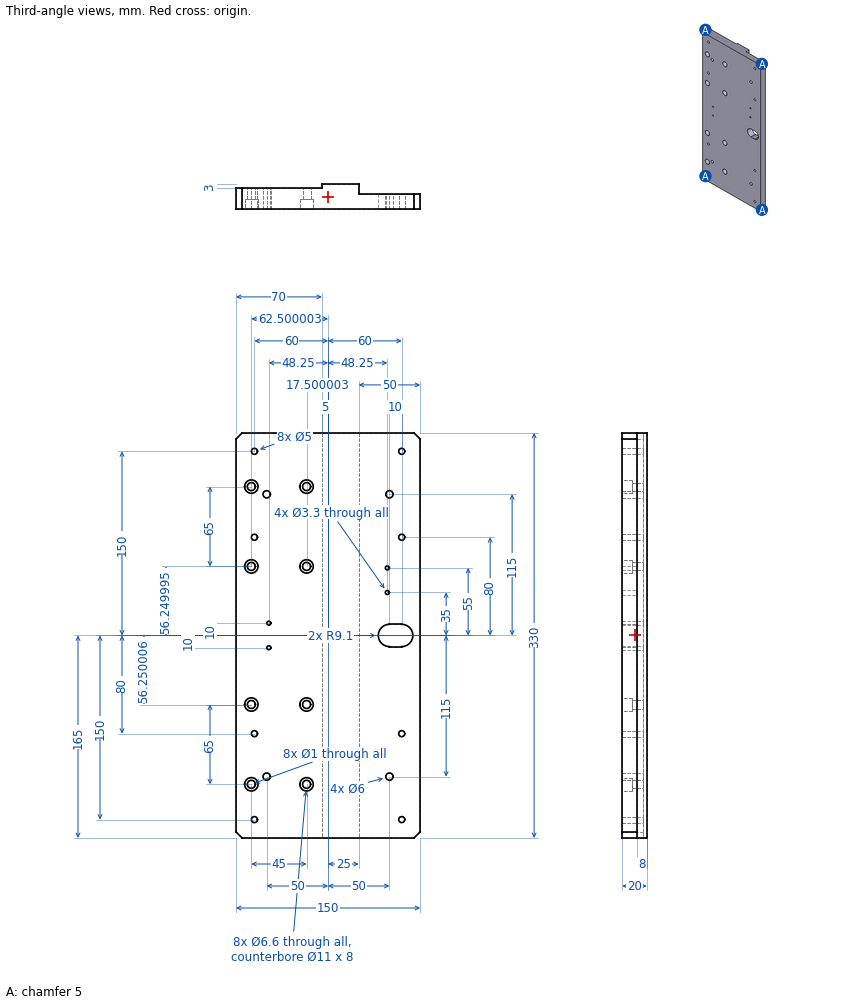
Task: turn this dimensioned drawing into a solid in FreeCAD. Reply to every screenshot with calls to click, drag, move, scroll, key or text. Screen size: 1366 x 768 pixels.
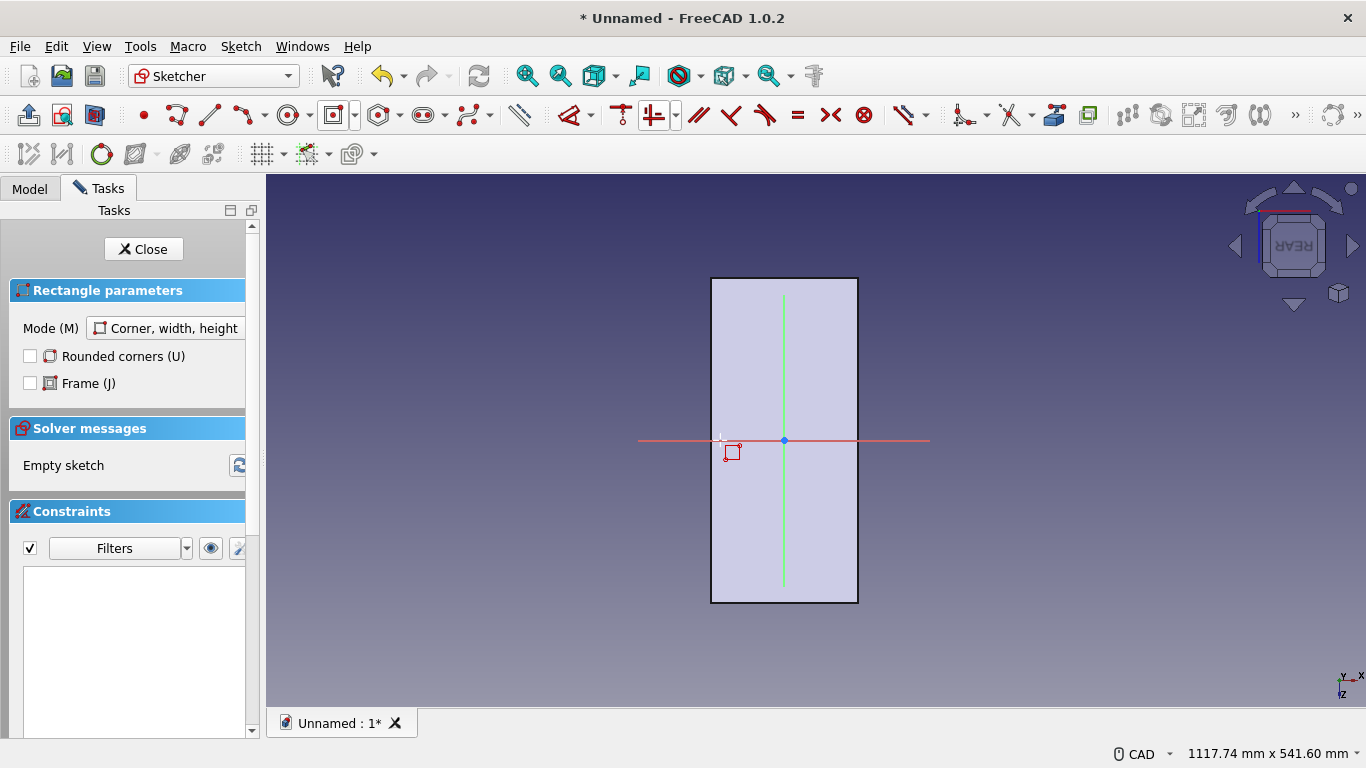
click(711, 278)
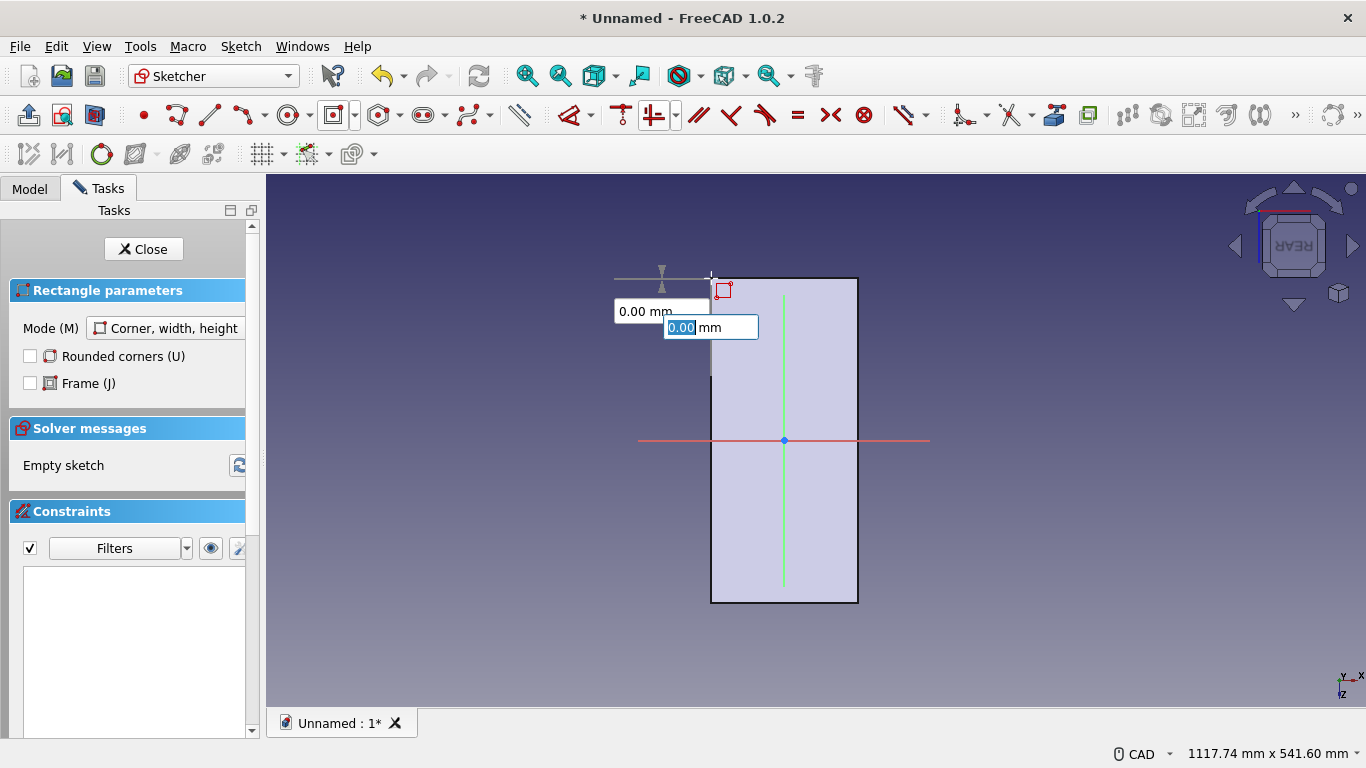
scroll(780, 603, up, 6)
move(777, 601)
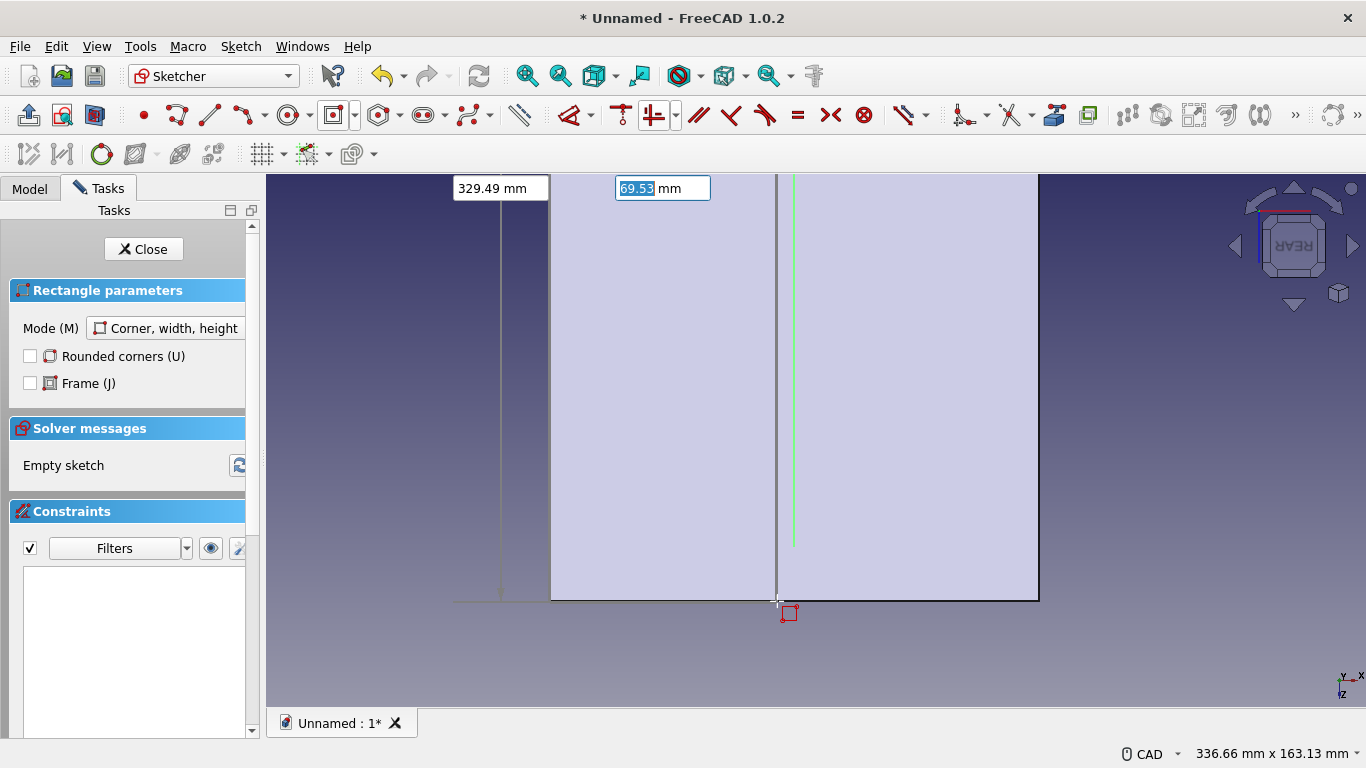
text(70)
key(Tab)
text(330)
key(Return)
key(Escape)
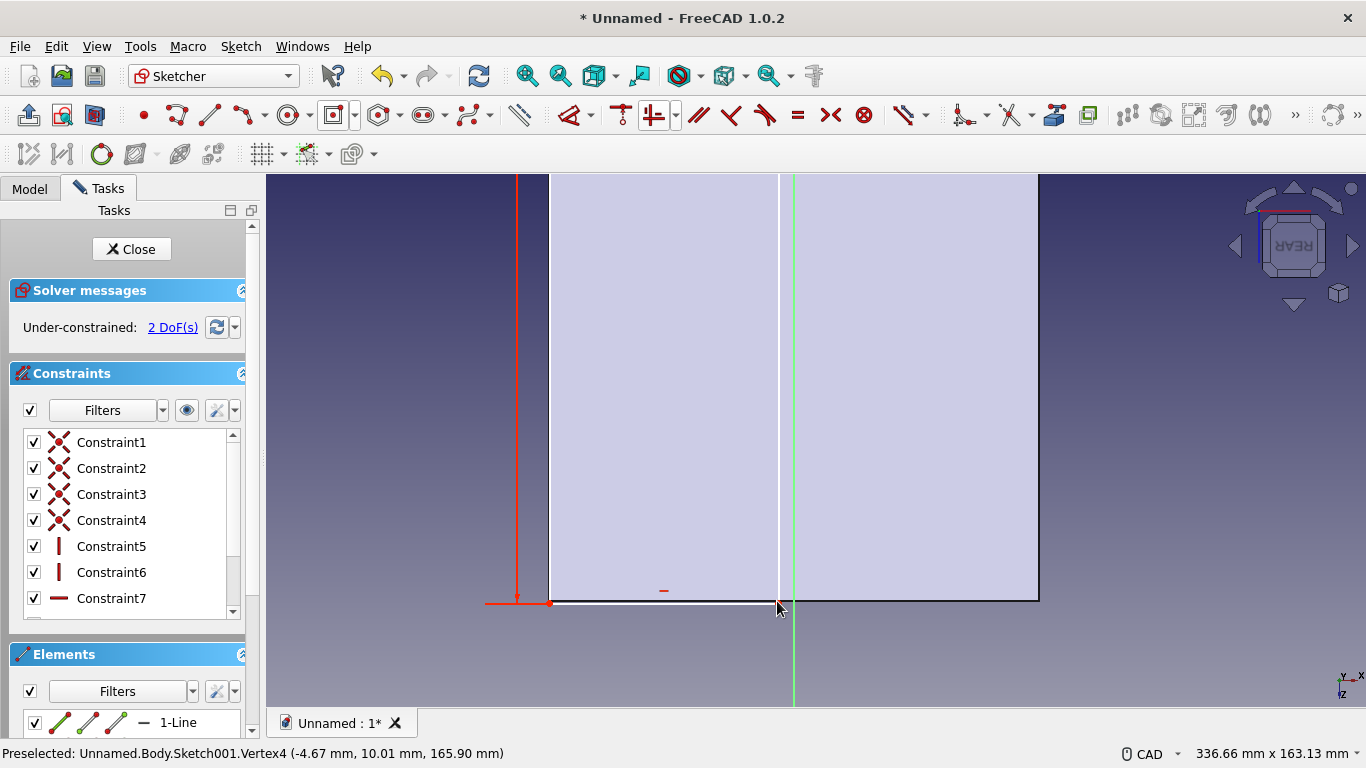
click(568, 116)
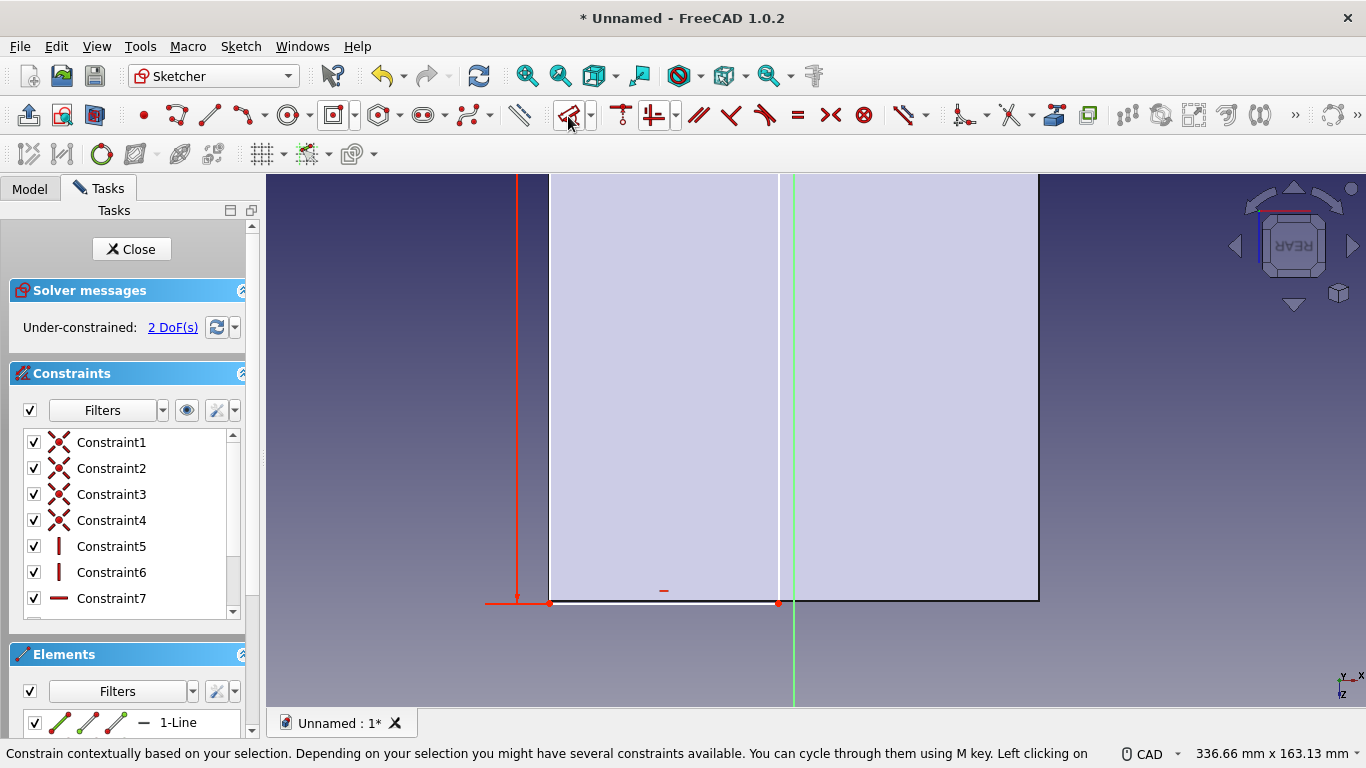
scroll(779, 604, up, 5)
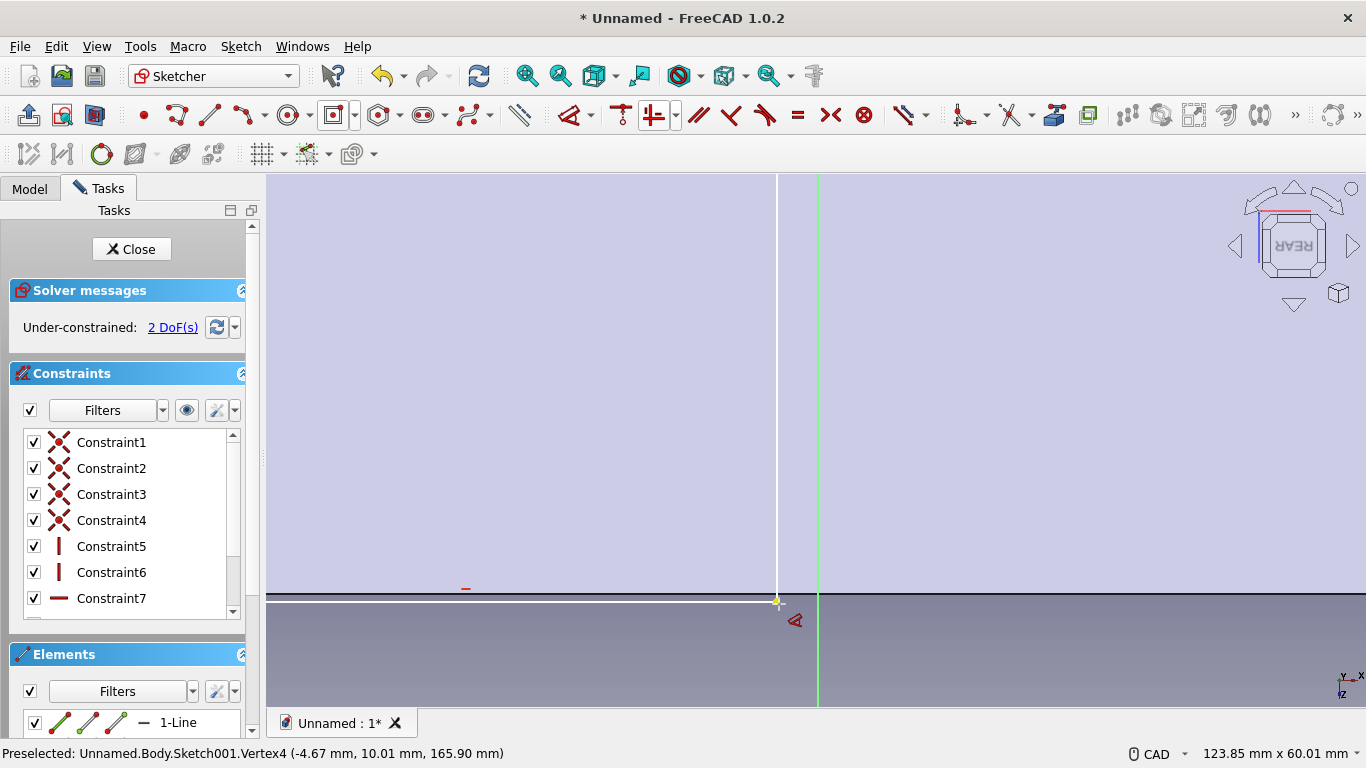
click(777, 602)
click(798, 636)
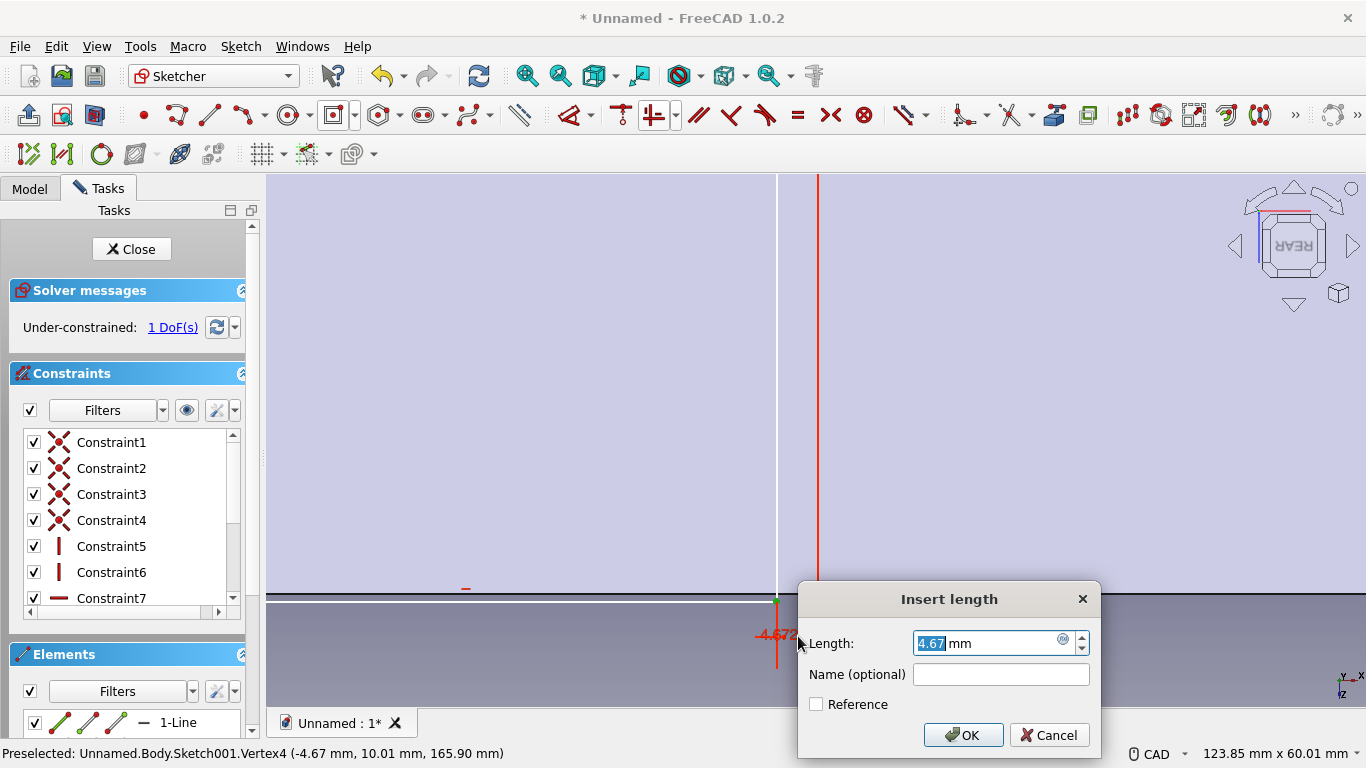
text(5)
key(Return)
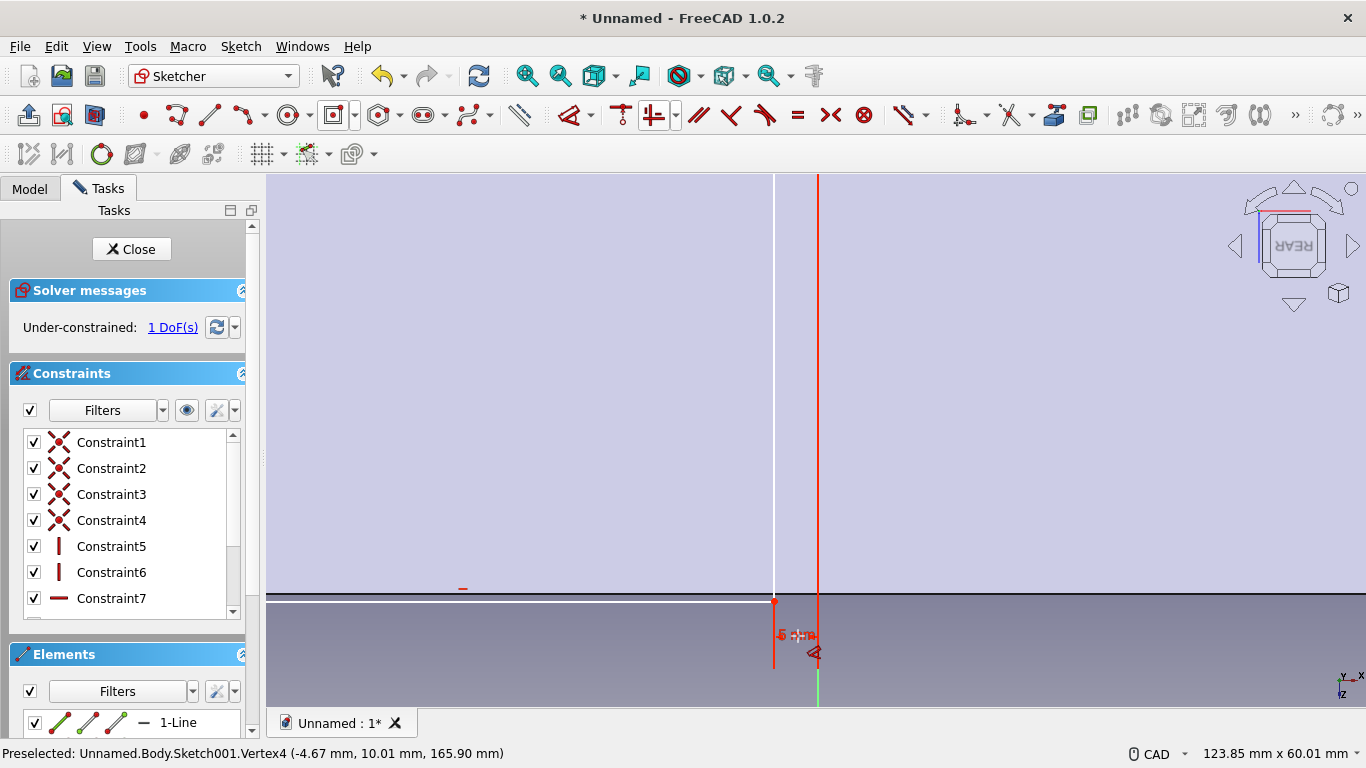
scroll(780, 604, down, 11)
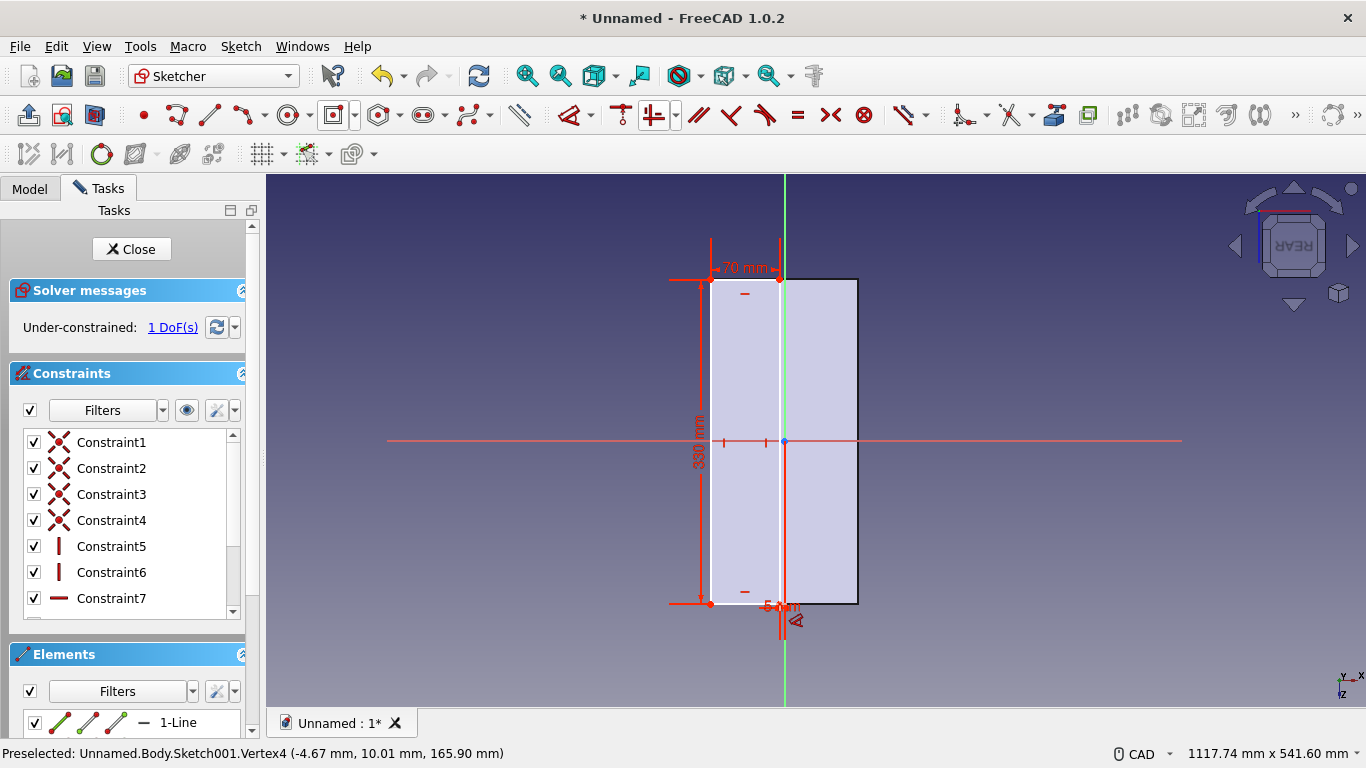
click(711, 280)
click(819, 360)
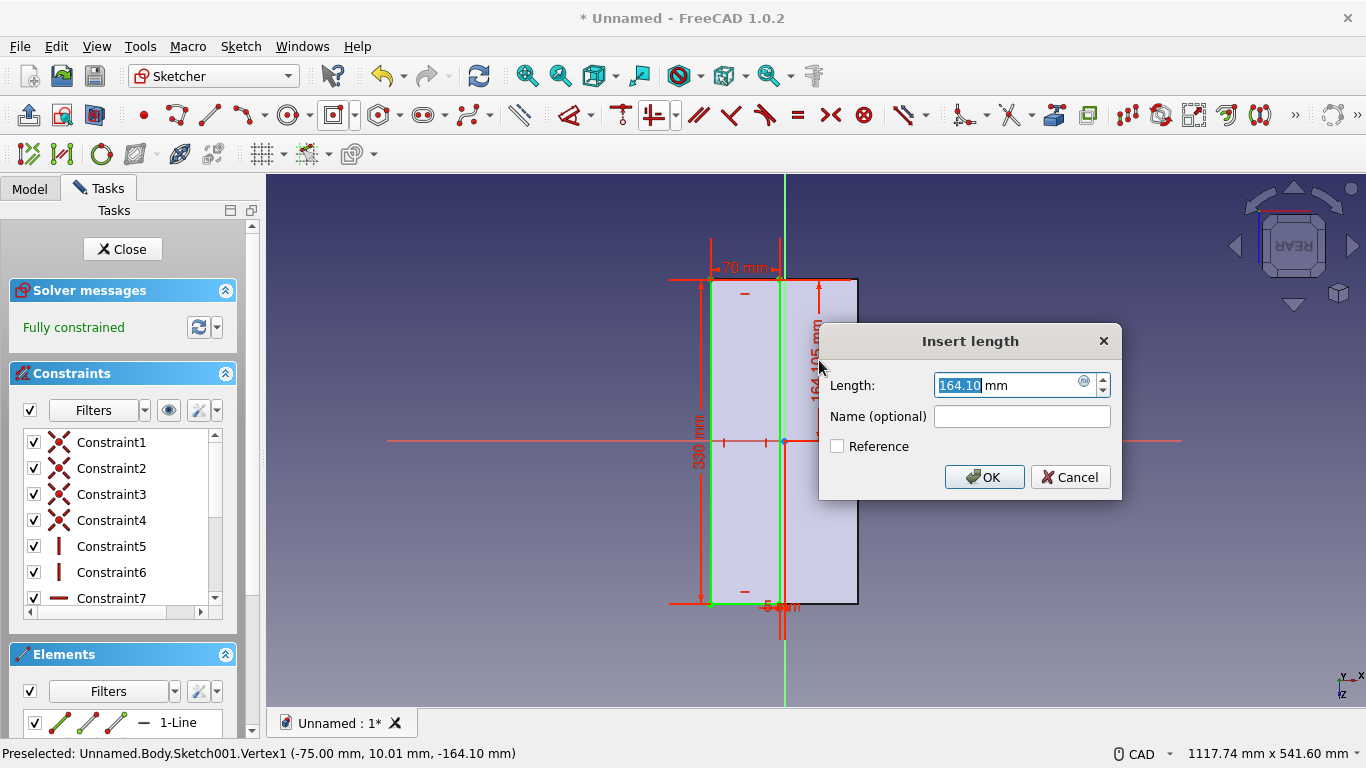
text(165)
key(Return)
key(Escape)